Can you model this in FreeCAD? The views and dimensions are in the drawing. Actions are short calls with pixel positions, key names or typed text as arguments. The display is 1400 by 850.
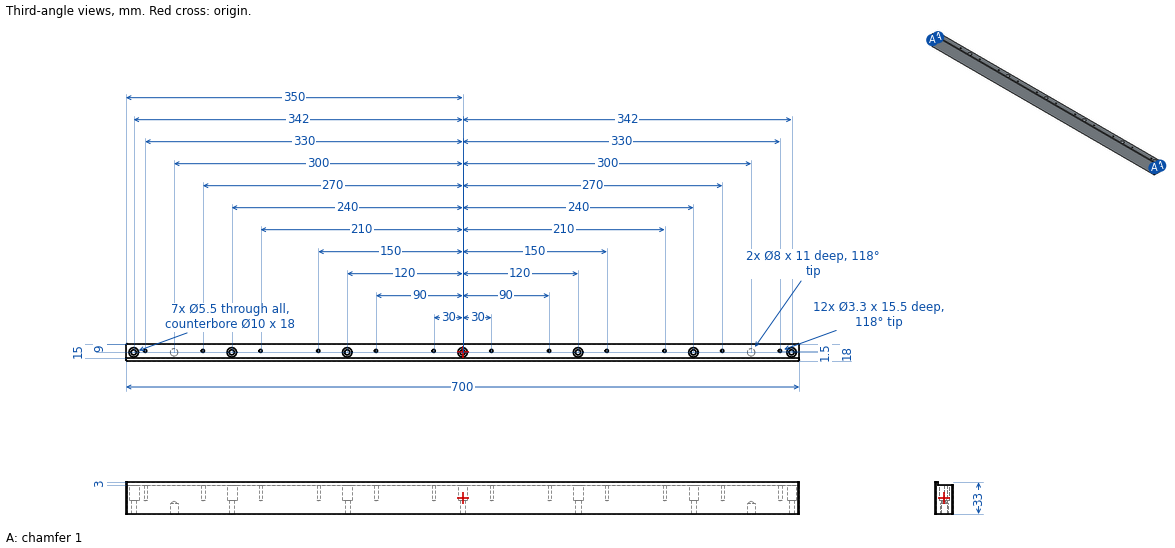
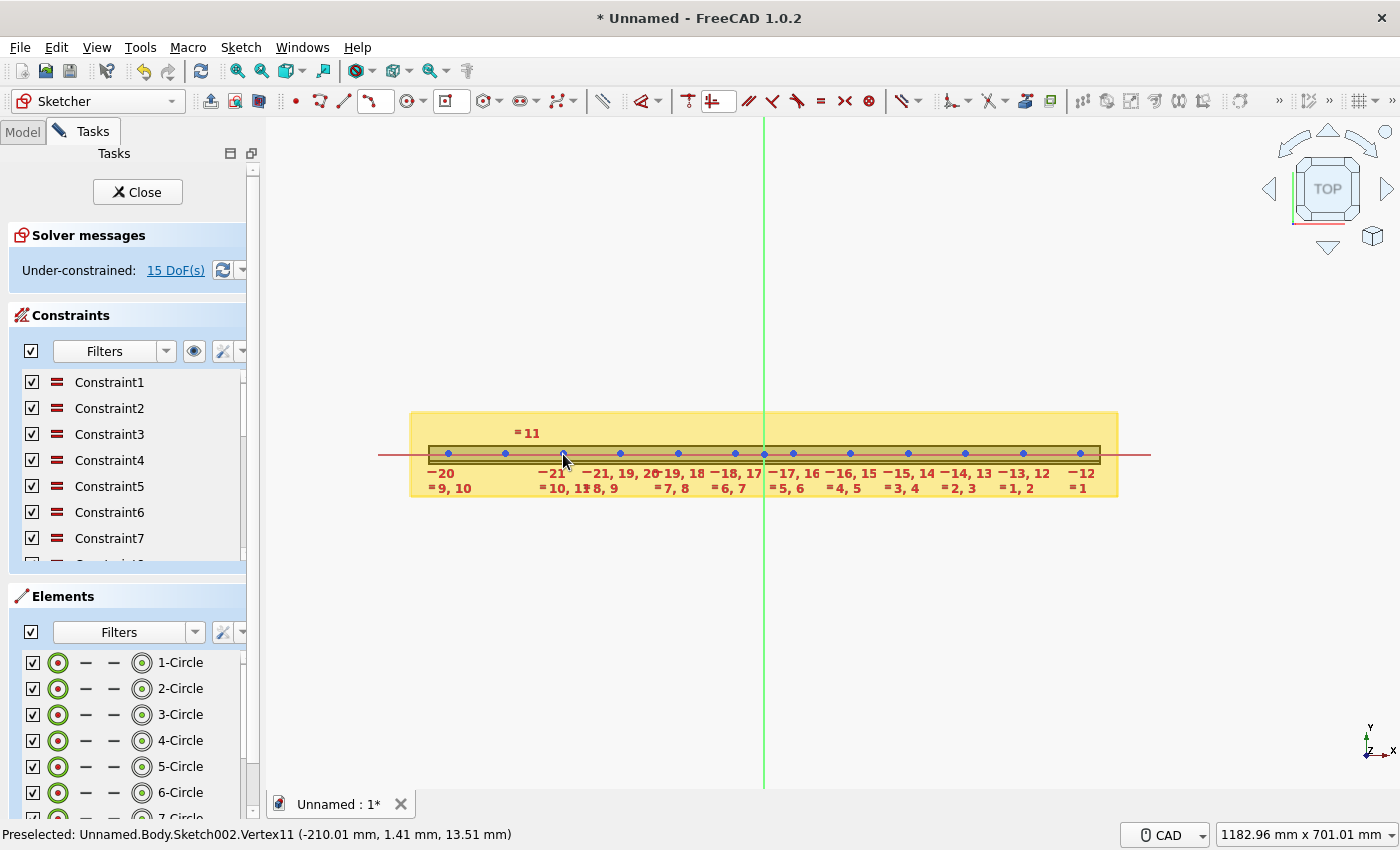
click(448, 453)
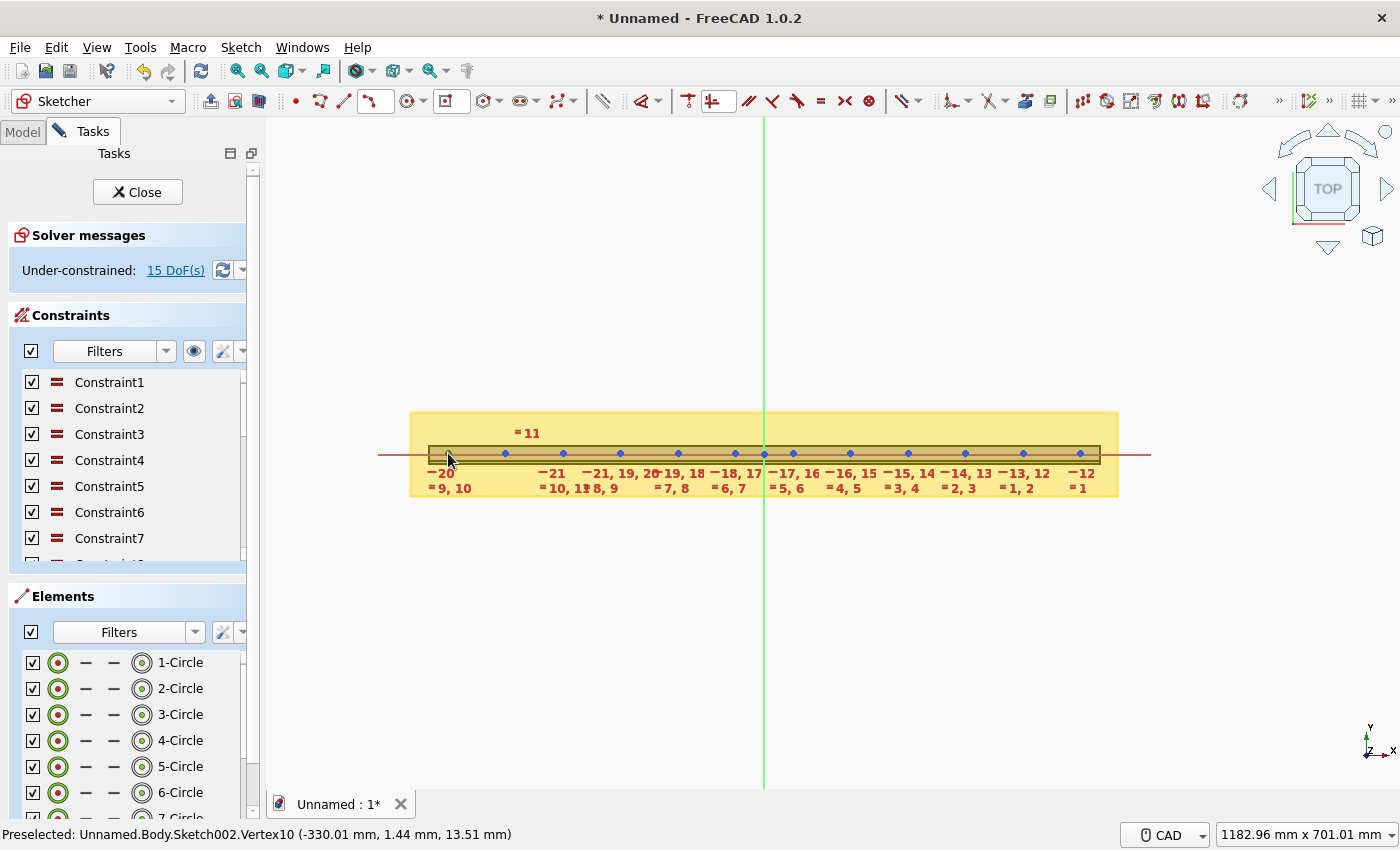
click(506, 454)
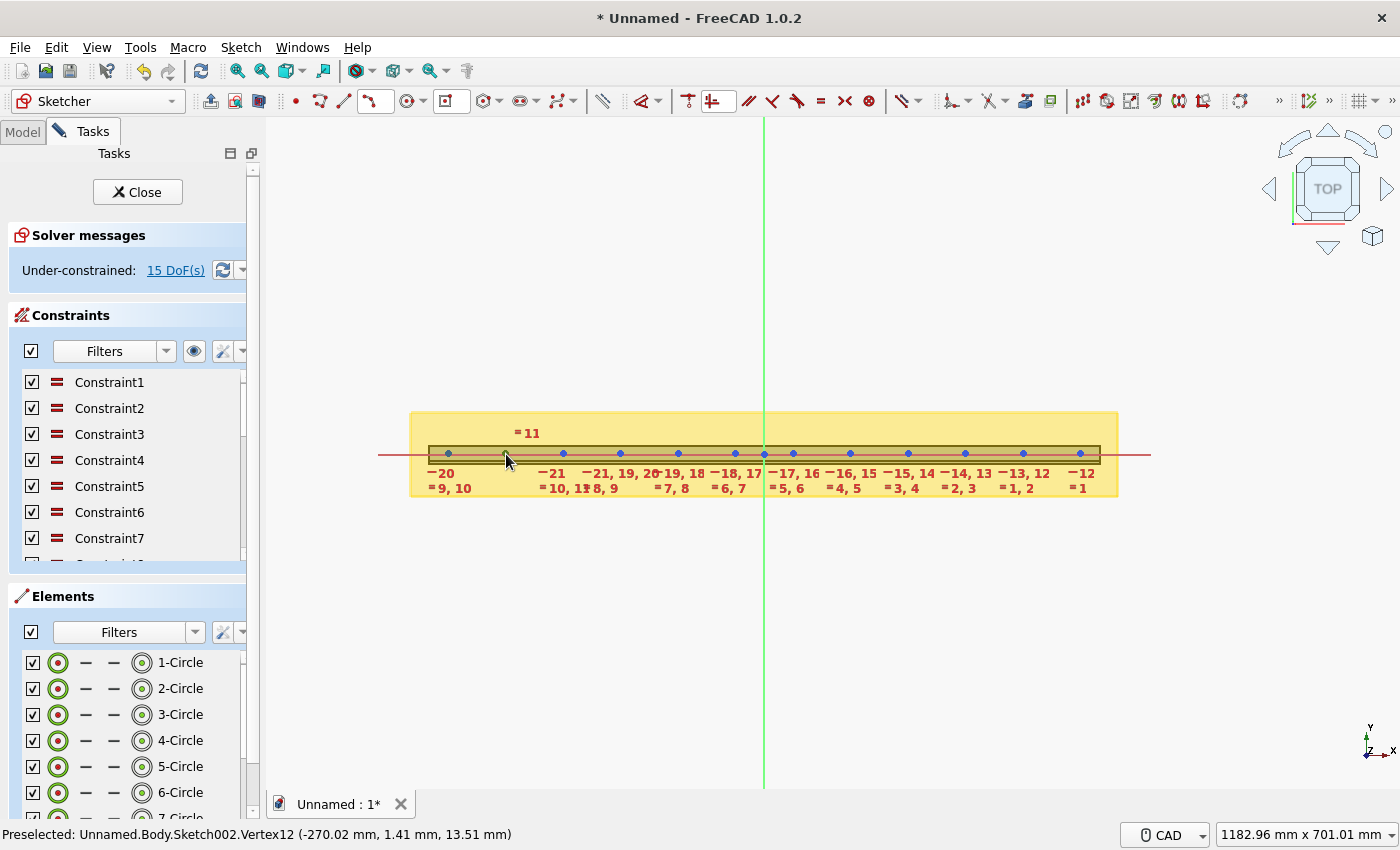
key(h)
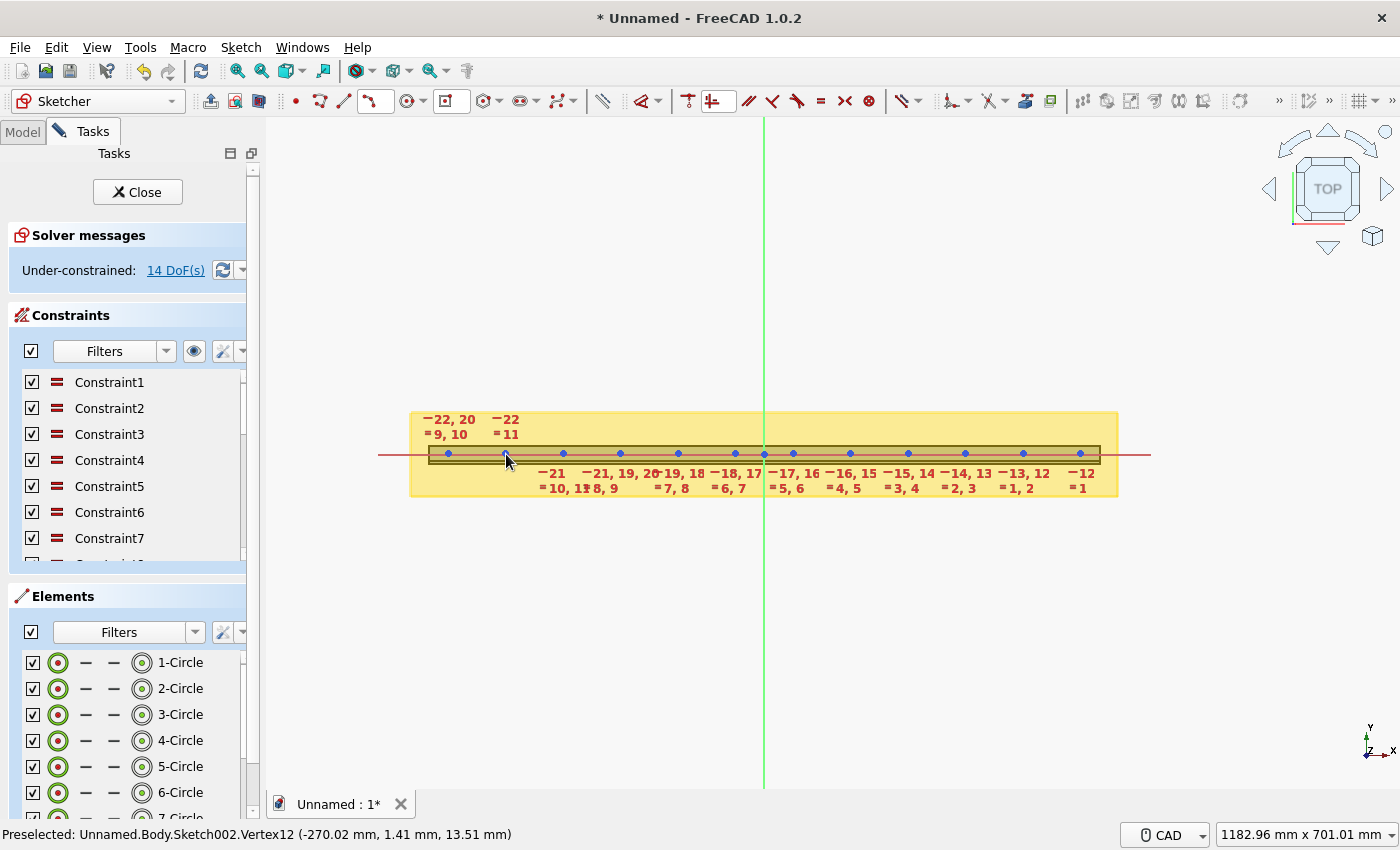
key(d)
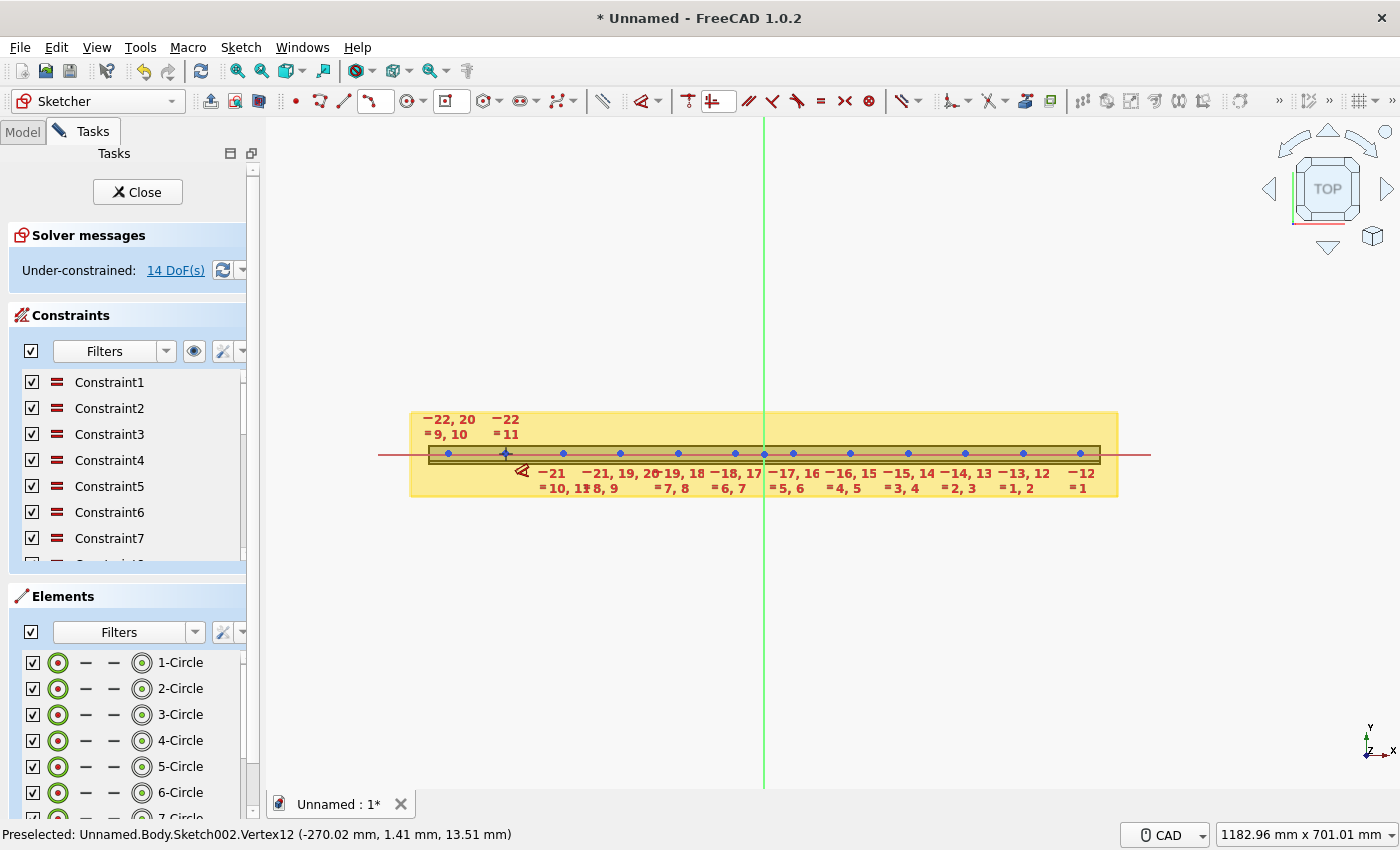
scroll(1081, 455, up, 13)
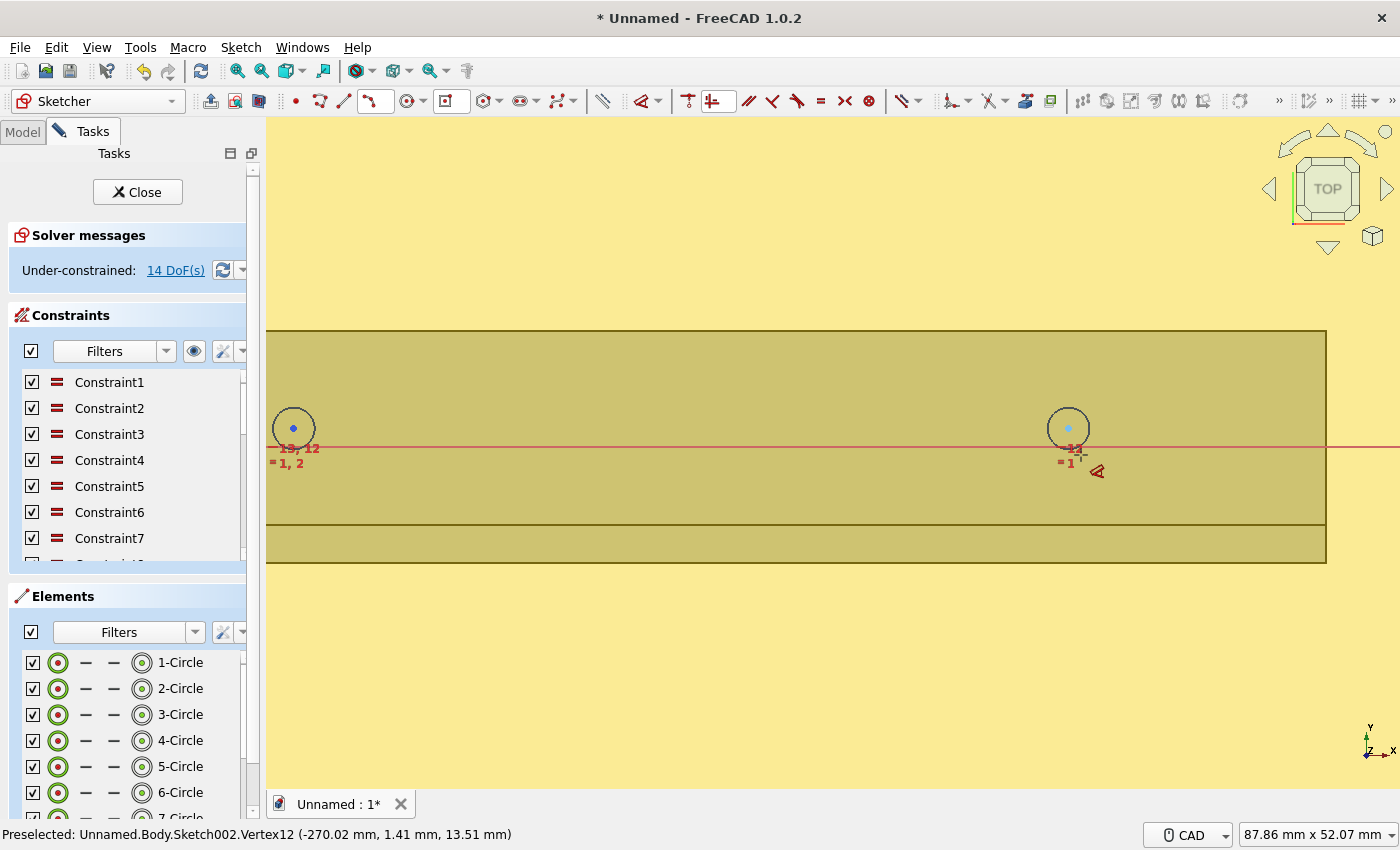
click(1068, 449)
click(1067, 481)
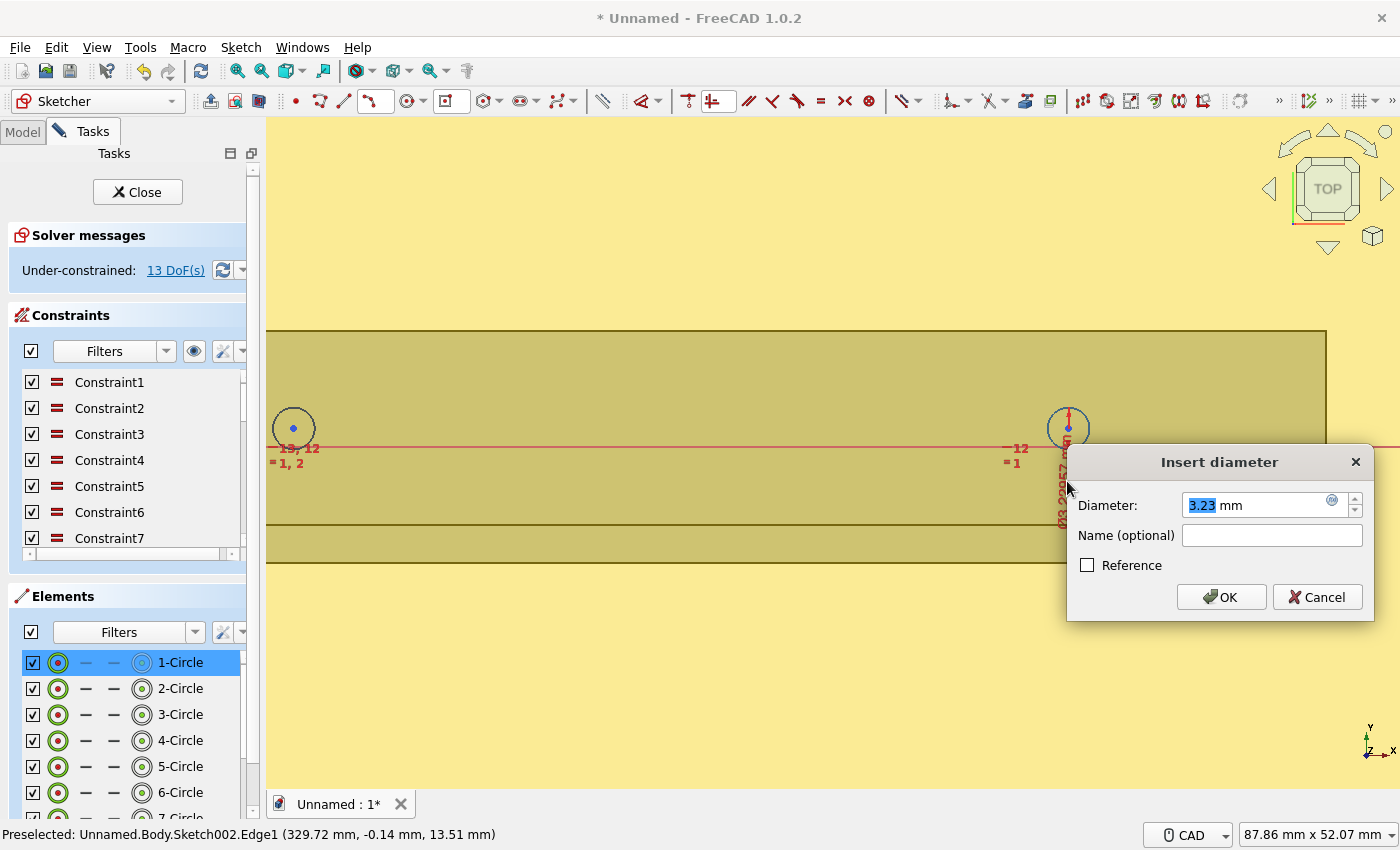
text(3.3)
key(Return)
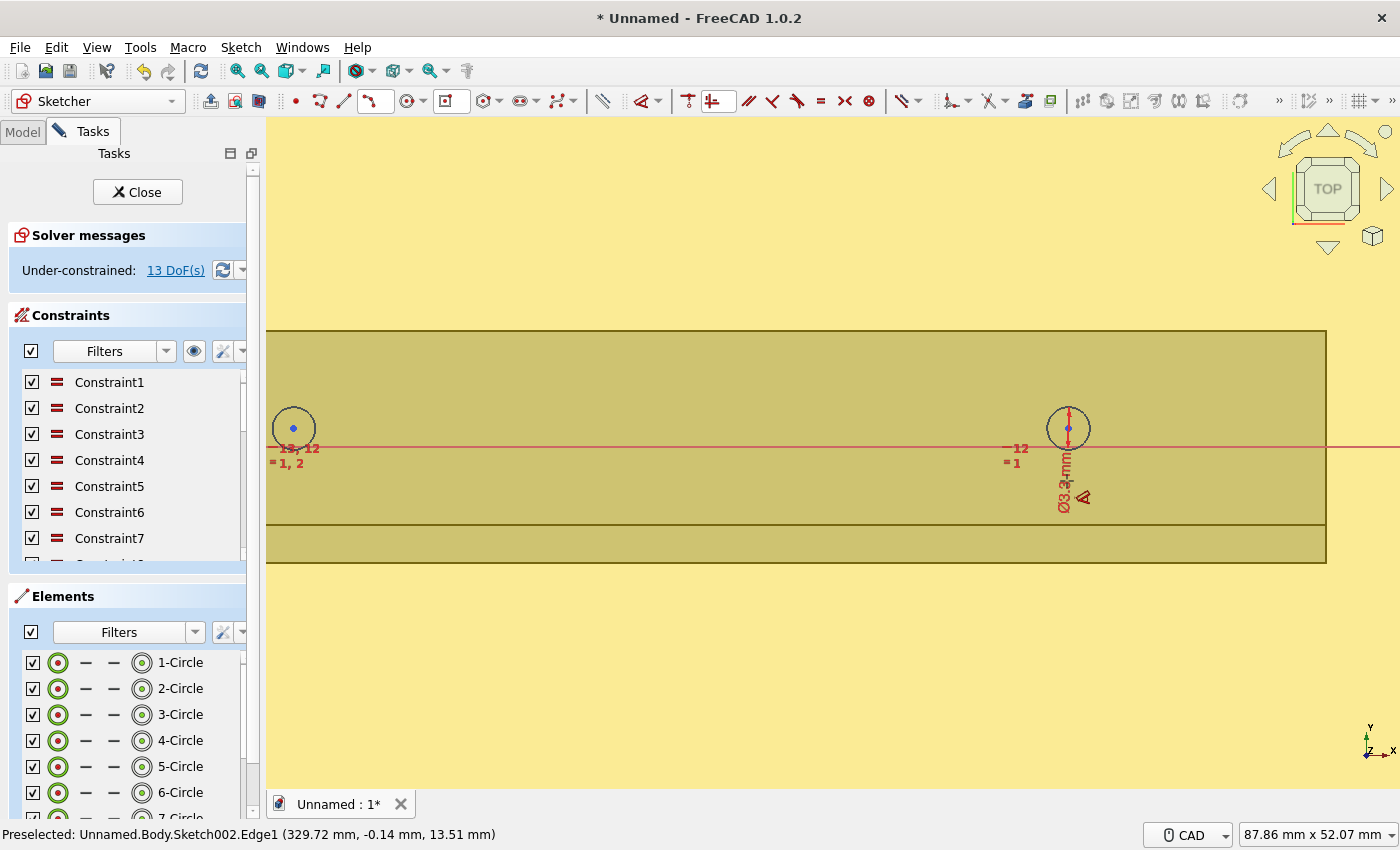
scroll(1082, 455, down, 13)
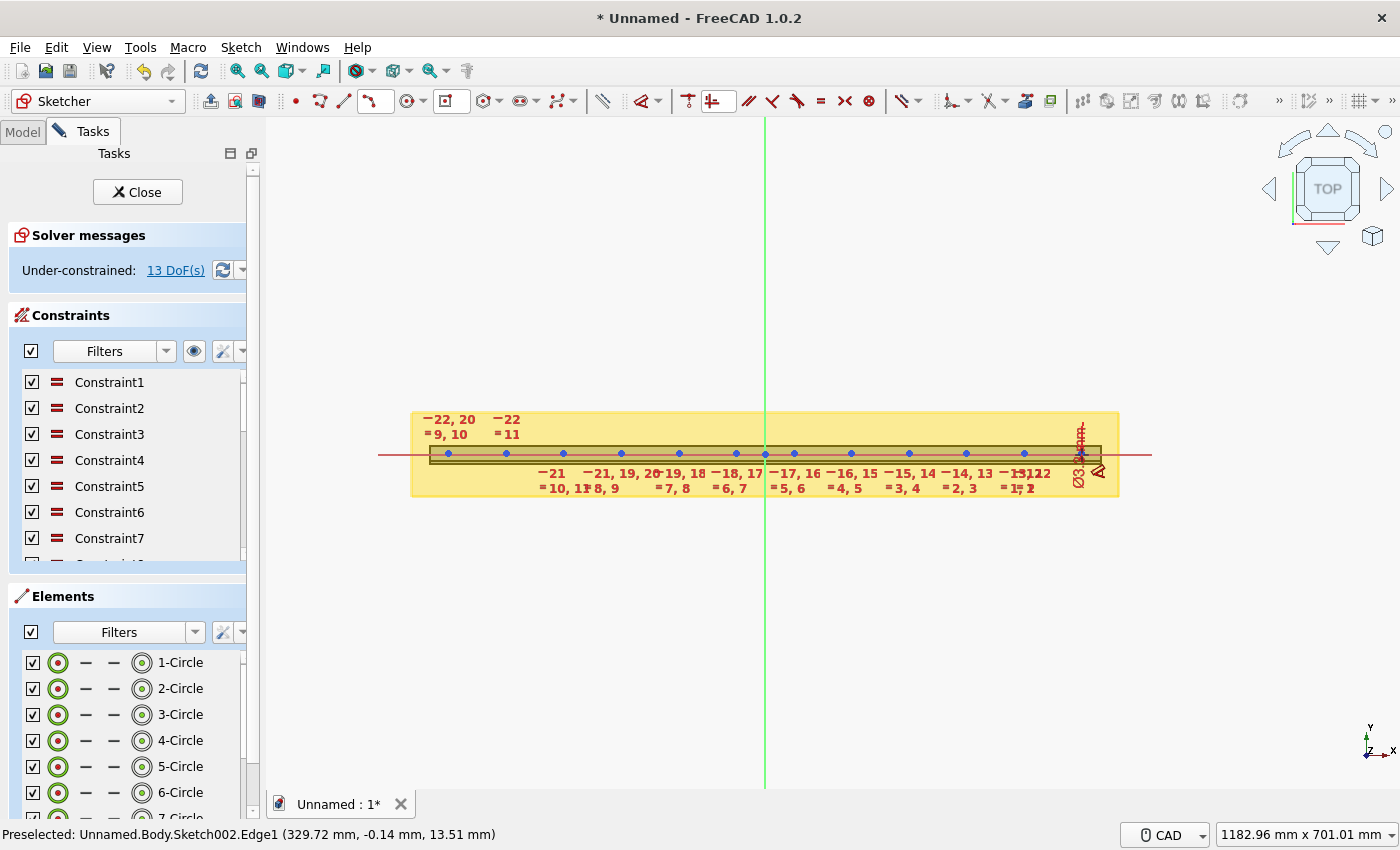
click(852, 453)
click(808, 489)